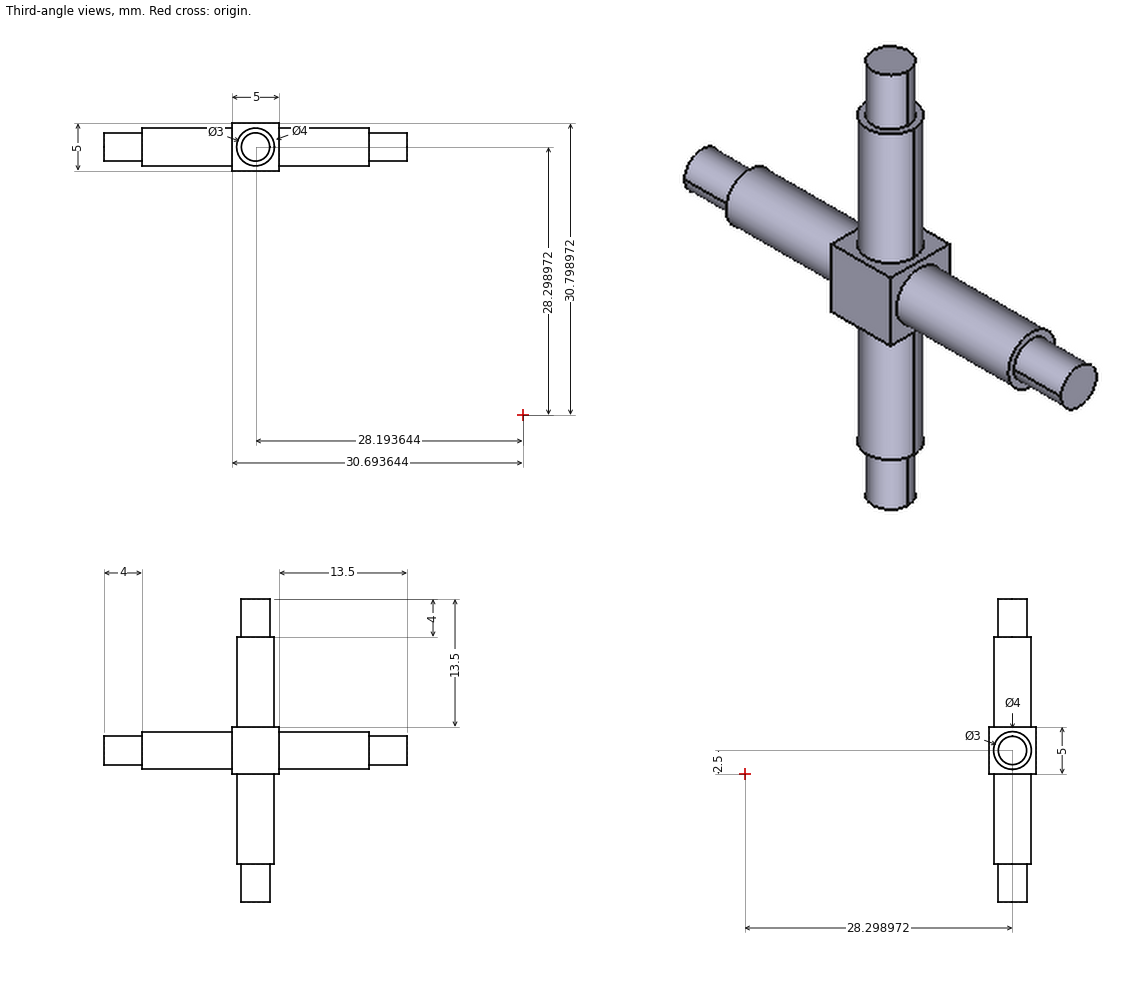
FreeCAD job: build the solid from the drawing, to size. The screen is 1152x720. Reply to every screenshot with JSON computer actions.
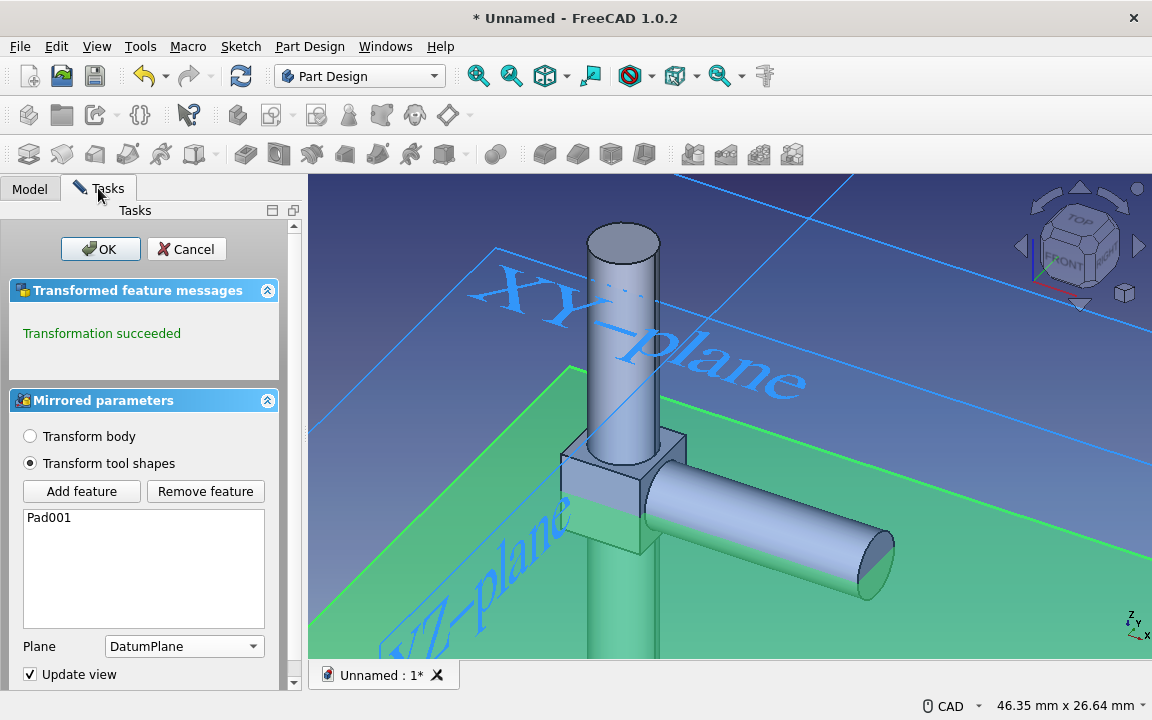
{"action": "left_click", "coordinate": [101, 249]}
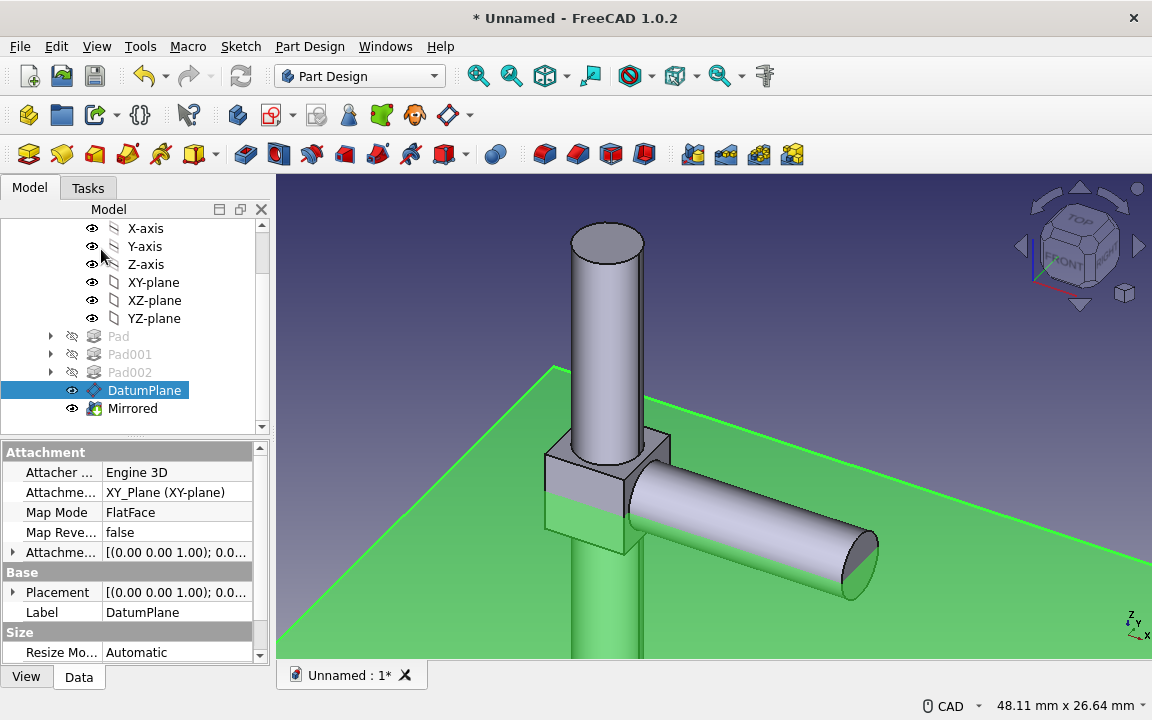
{"action": "left_click", "coordinate": [117, 390]}
{"action": "key", "text": "space"}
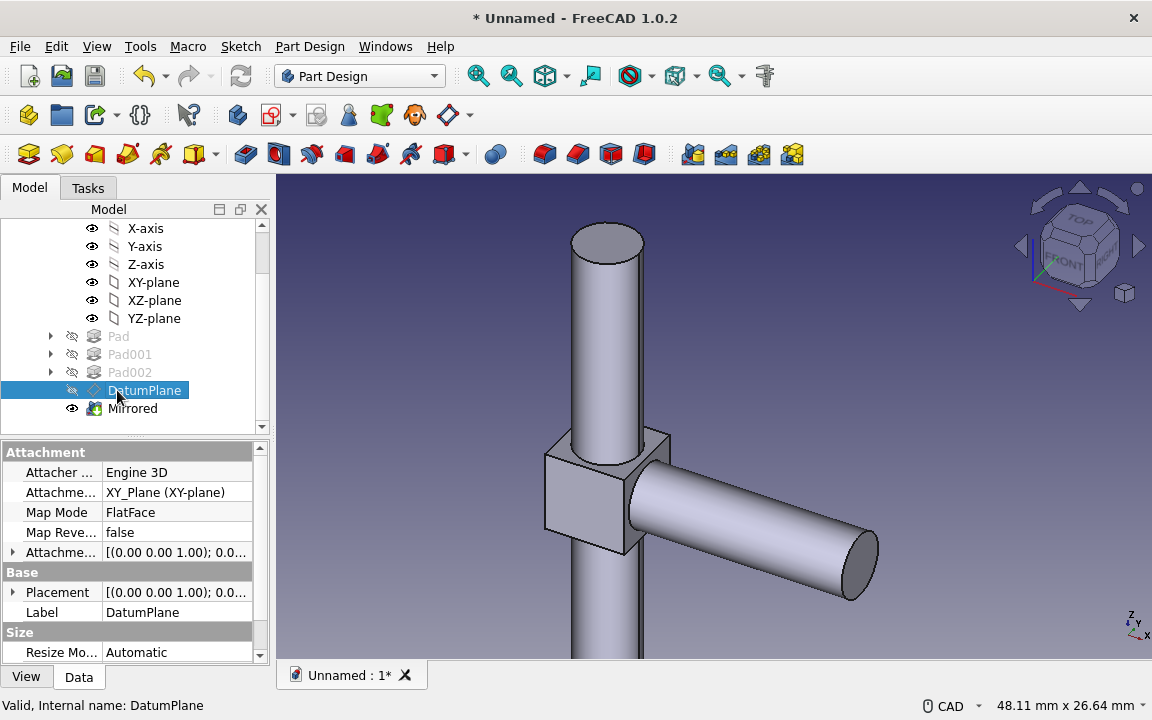
{"action": "key", "text": "v f"}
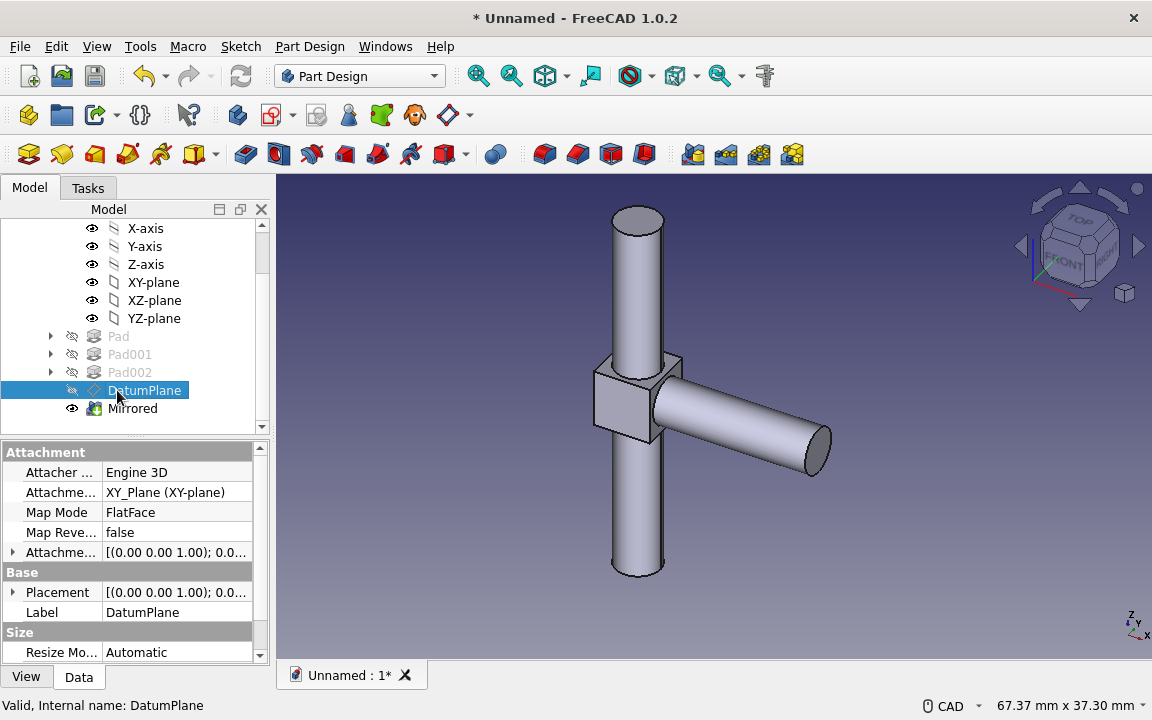
{"action": "scroll", "coordinate": [161, 314], "scroll_direction": "down", "scroll_amount": 3}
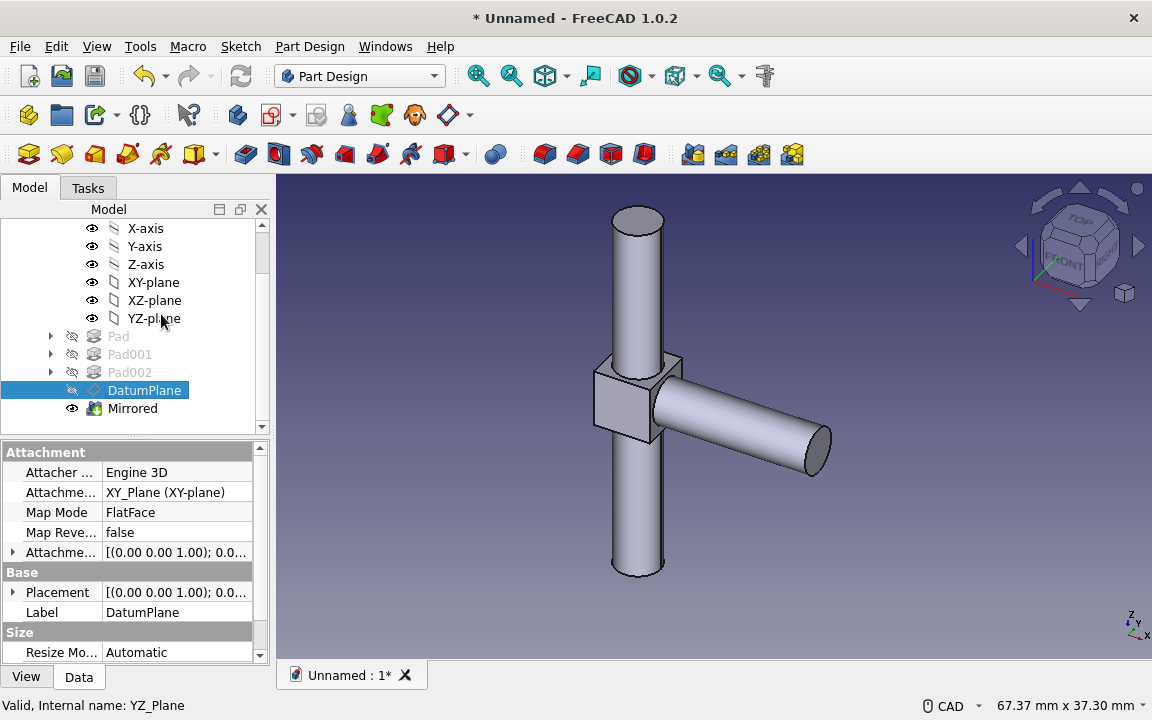
{"action": "scroll", "coordinate": [161, 314], "scroll_direction": "up", "scroll_amount": 15}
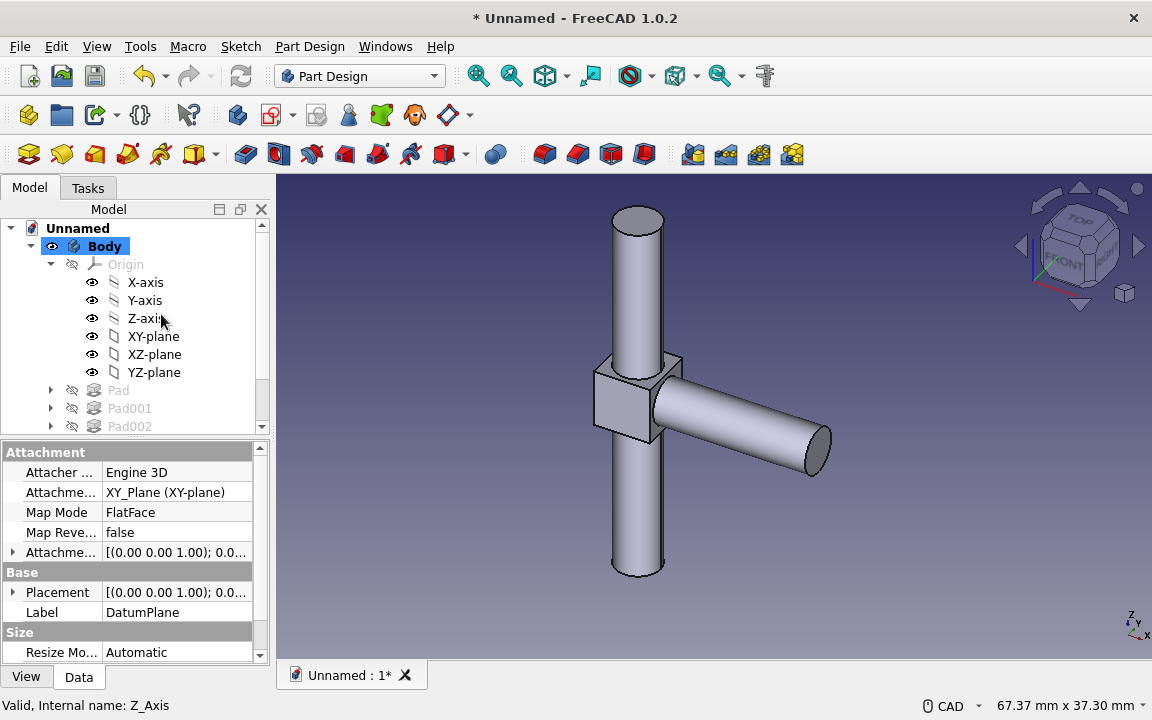
{"action": "left_click", "coordinate": [137, 372]}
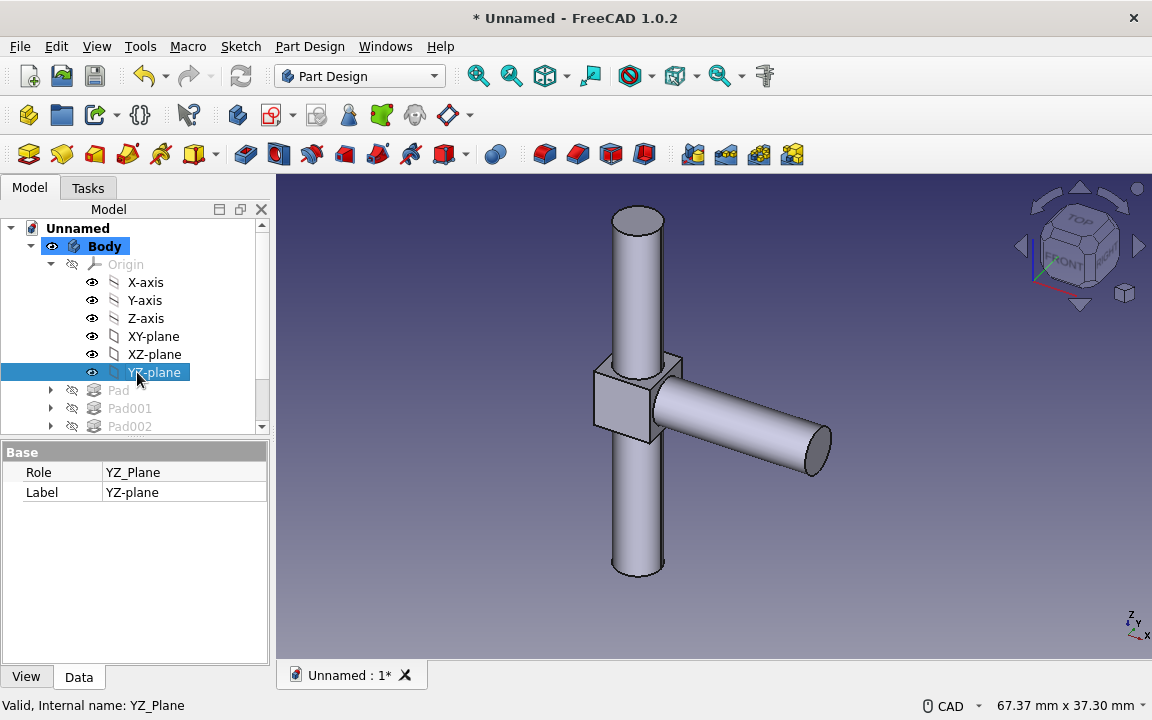
{"action": "left_click", "coordinate": [448, 116]}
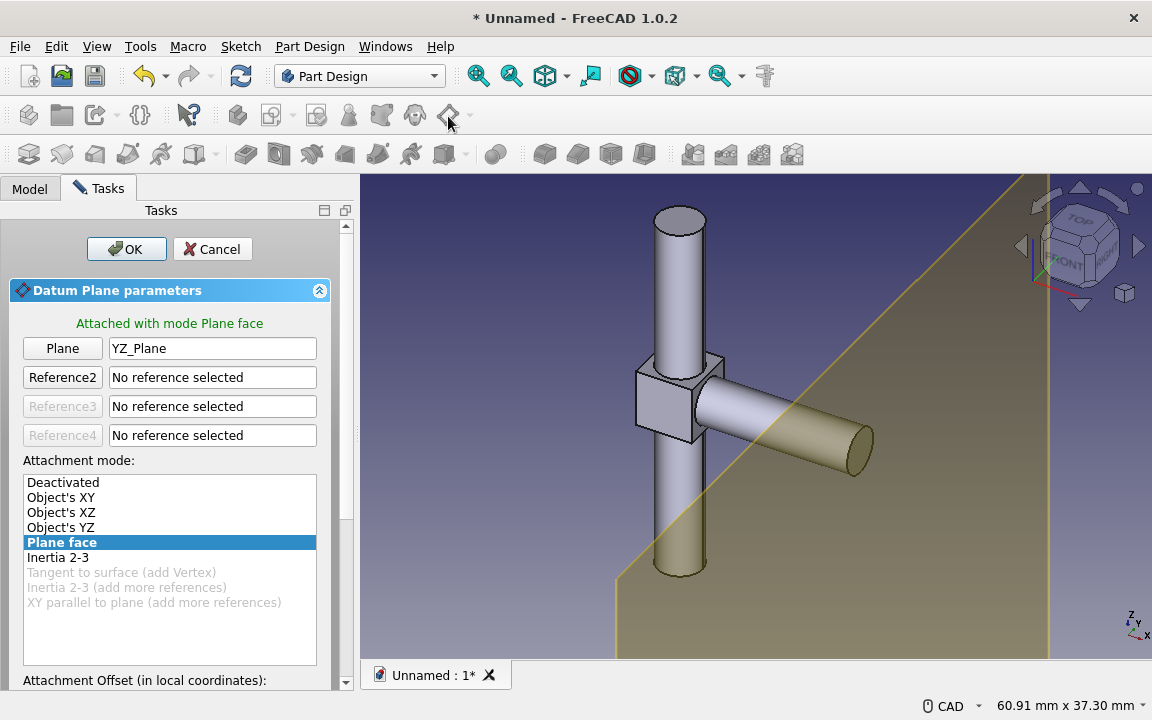
{"action": "scroll", "coordinate": [346, 455], "scroll_direction": "down", "scroll_amount": 3}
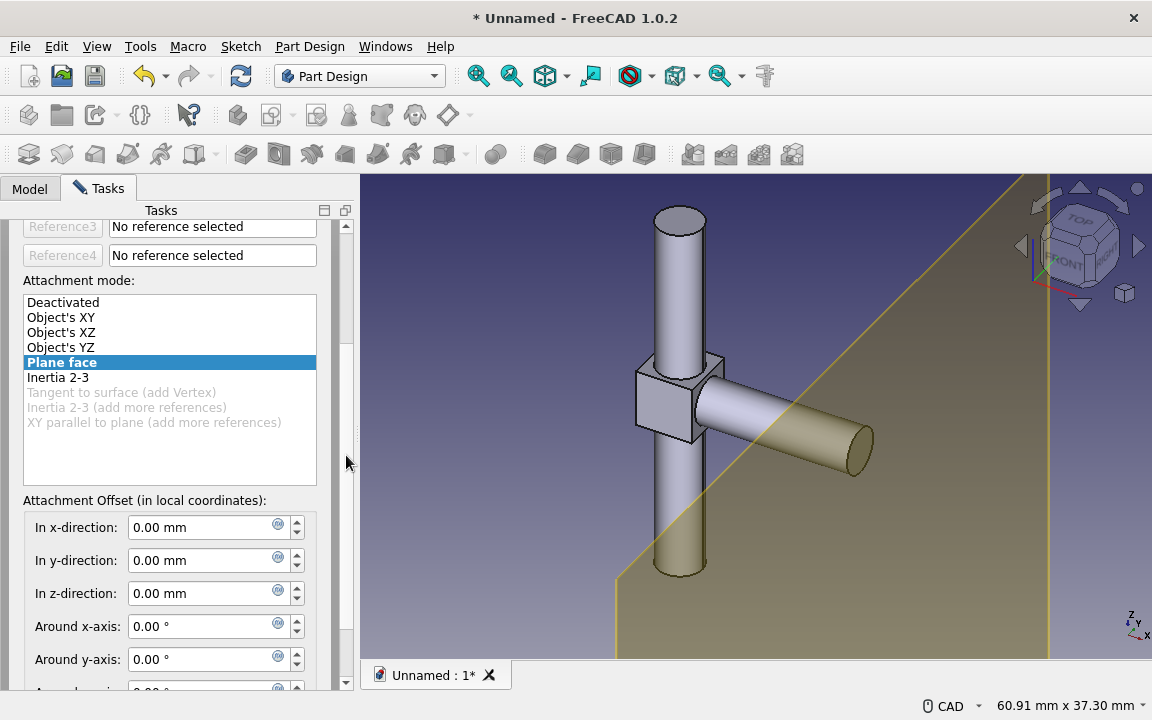
{"action": "triple_click", "coordinate": [210, 594]}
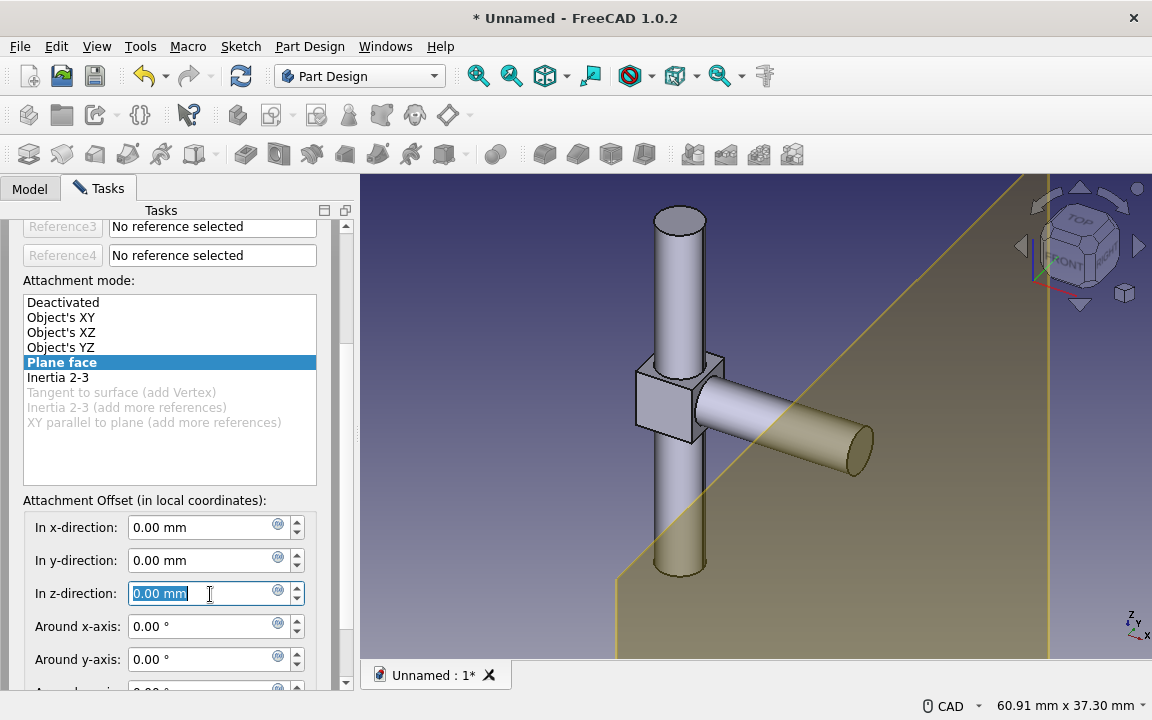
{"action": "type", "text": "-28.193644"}
{"action": "key", "text": "Tab"}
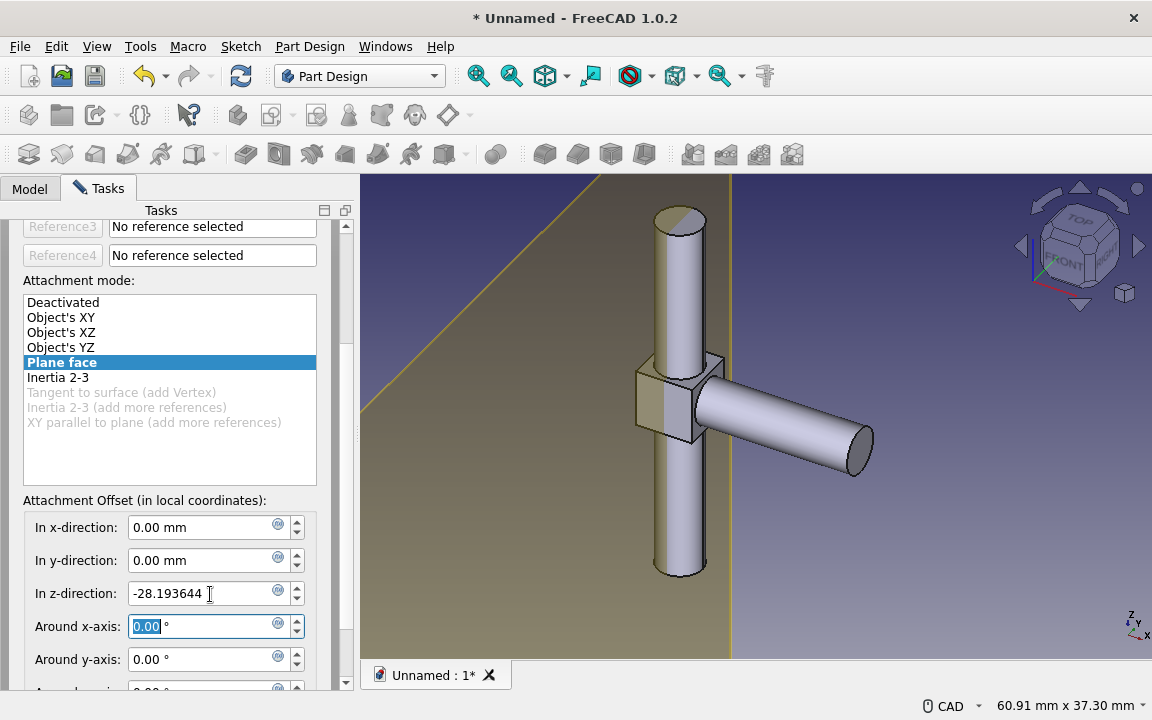
{"action": "scroll", "coordinate": [346, 455], "scroll_direction": "up", "scroll_amount": 4}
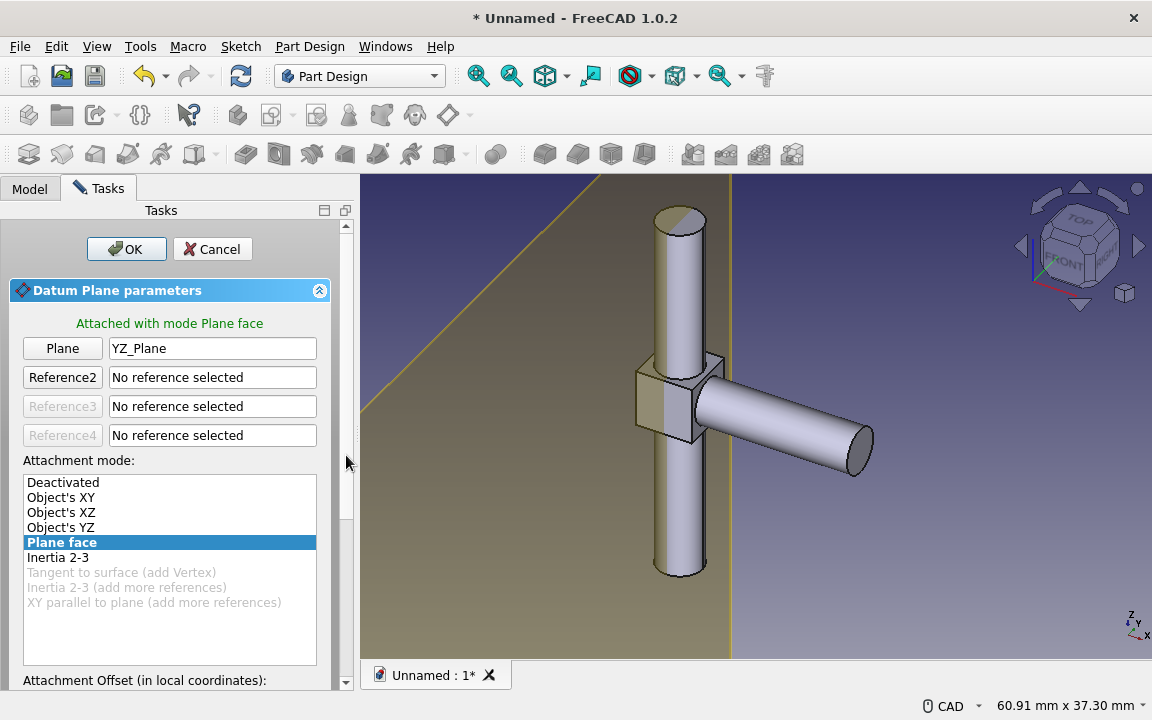
{"action": "left_click", "coordinate": [127, 249]}